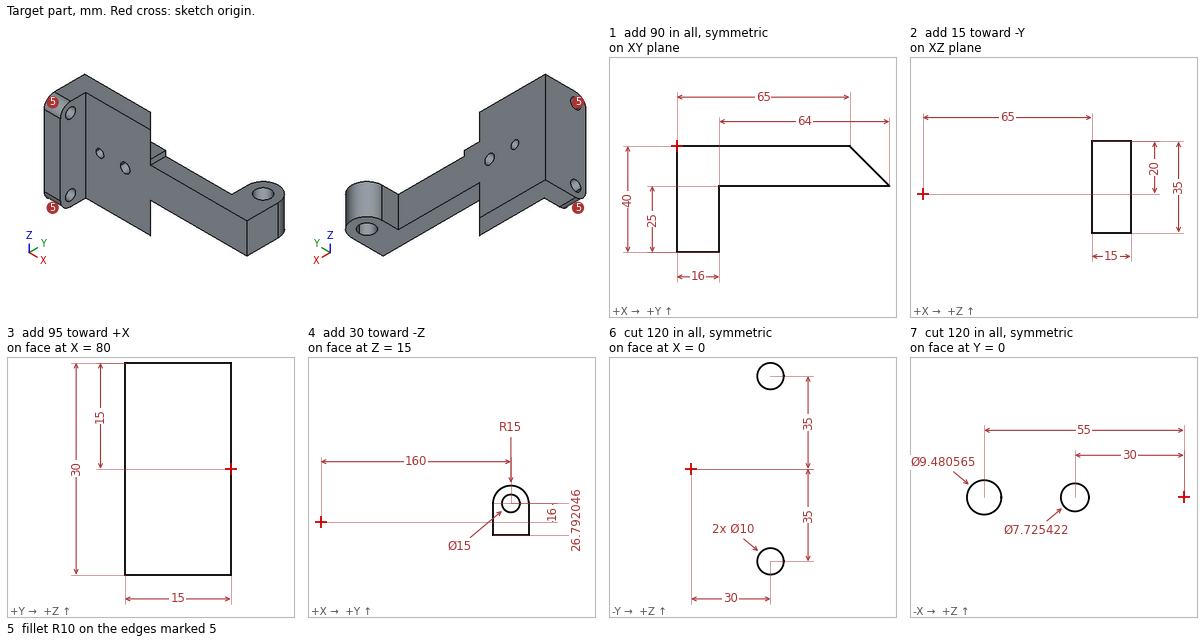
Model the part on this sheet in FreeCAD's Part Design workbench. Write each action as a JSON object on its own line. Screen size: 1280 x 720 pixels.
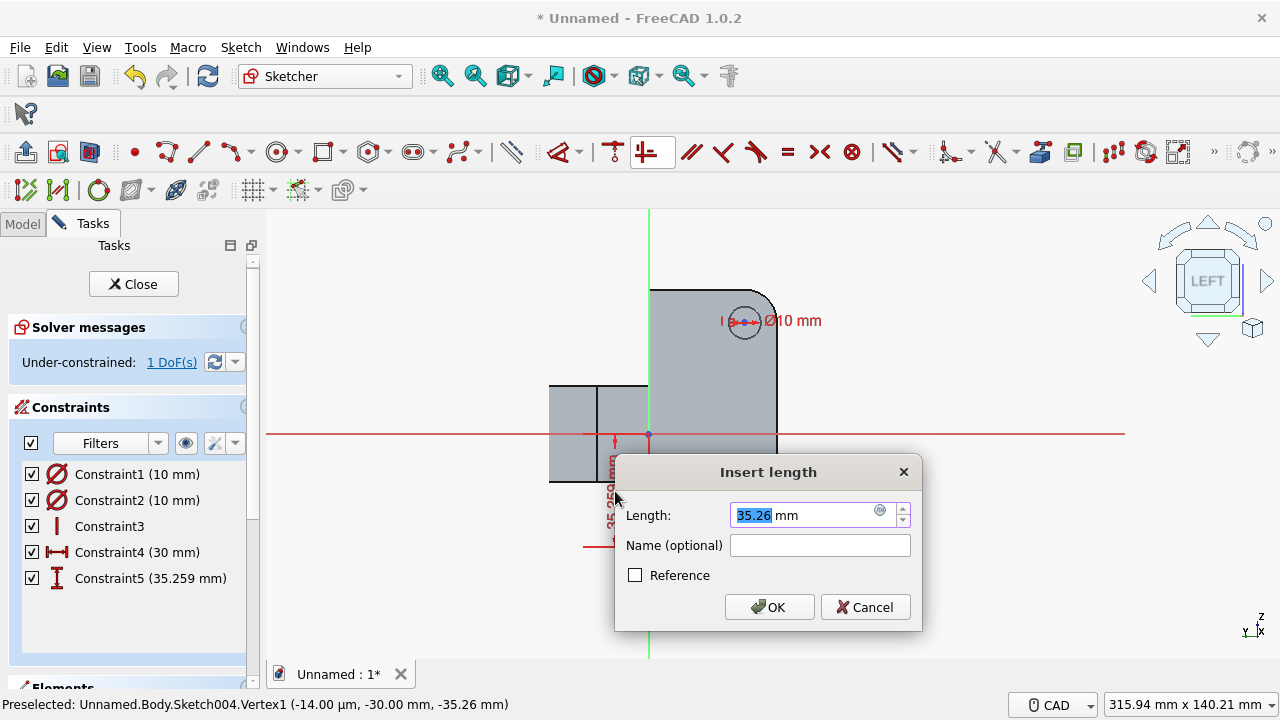
{"action": "type", "text": "35"}
{"action": "key", "text": "Return"}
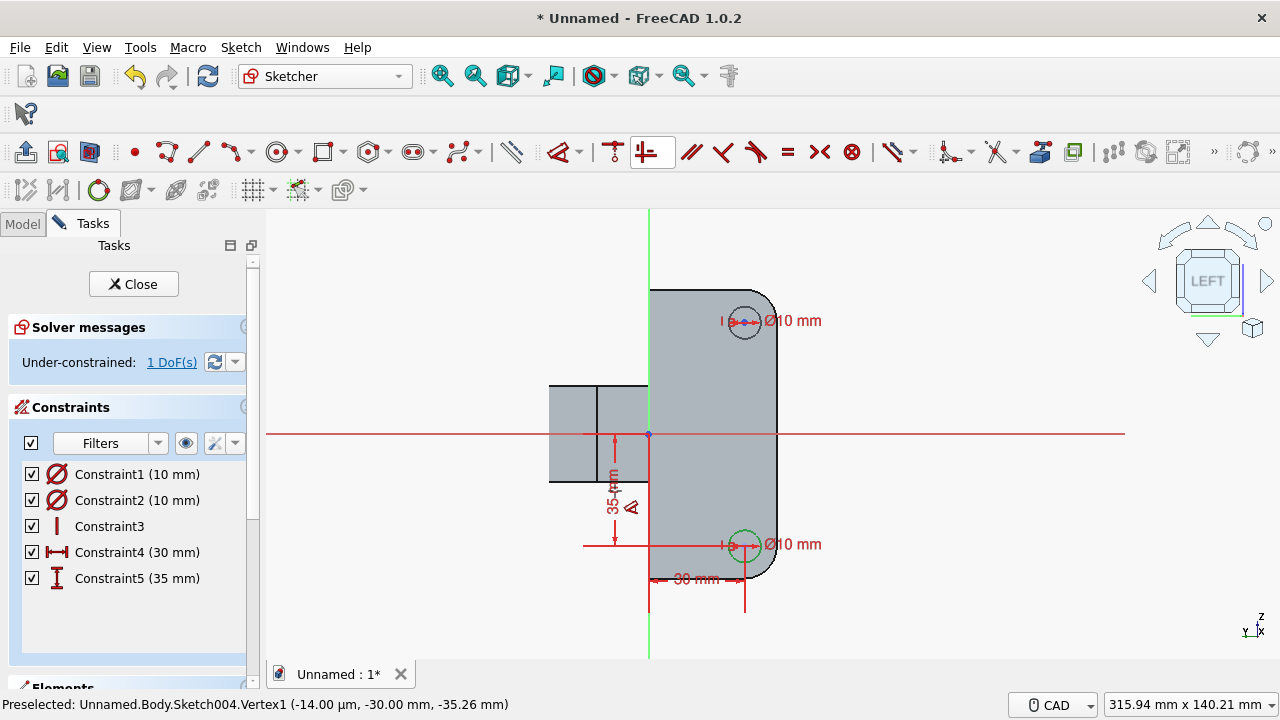
{"action": "left_click", "coordinate": [745, 323]}
{"action": "left_click", "coordinate": [615, 378]}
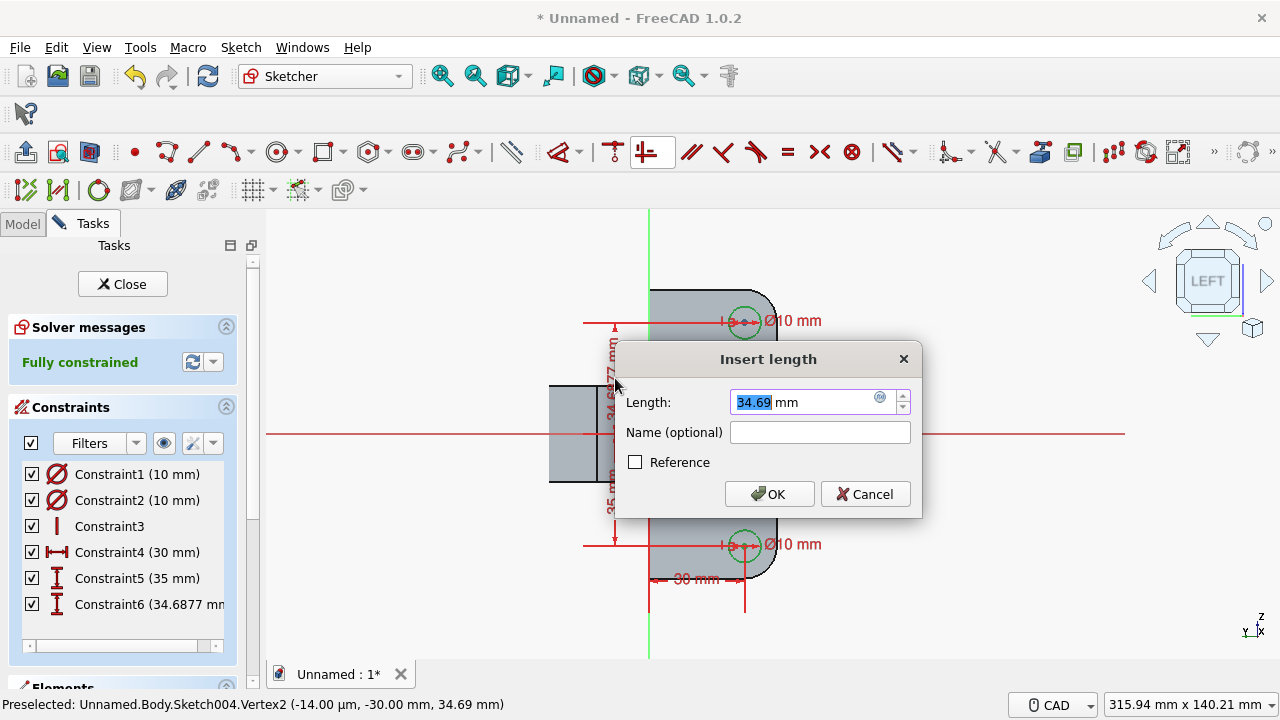
{"action": "type", "text": "35"}
{"action": "key", "text": "Return"}
{"action": "key", "text": "Escape"}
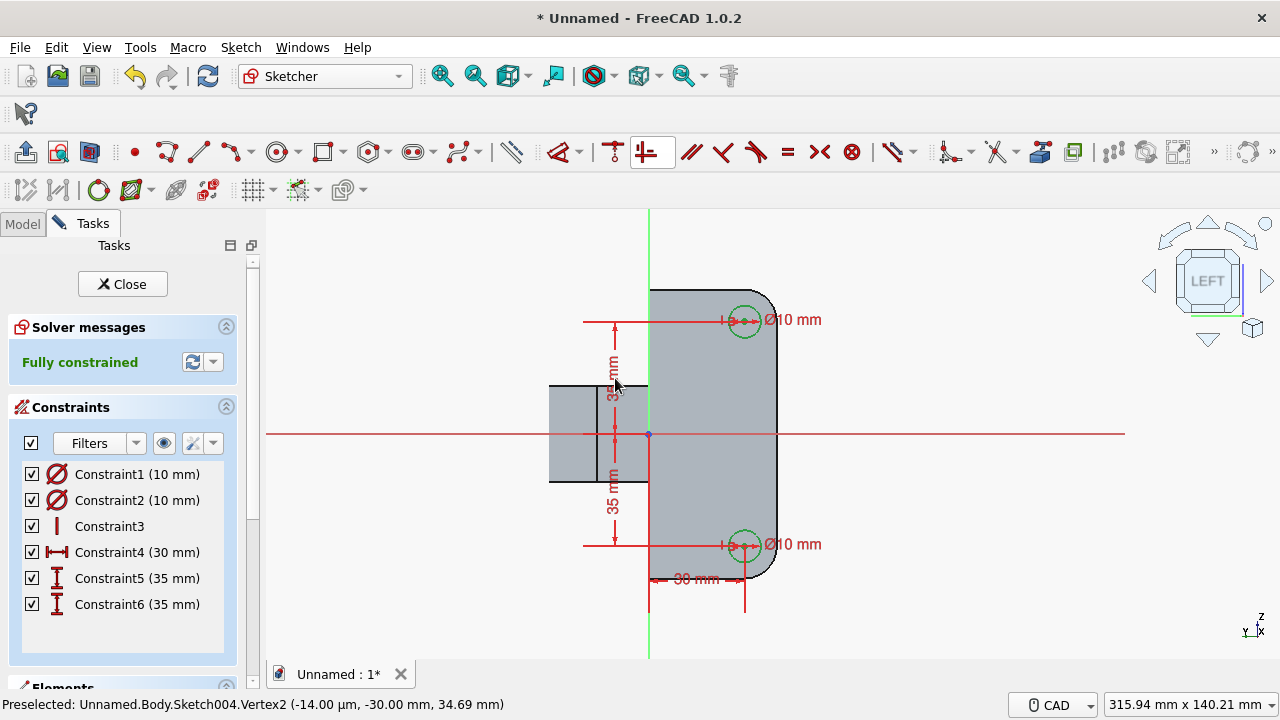
{"action": "left_click", "coordinate": [123, 284]}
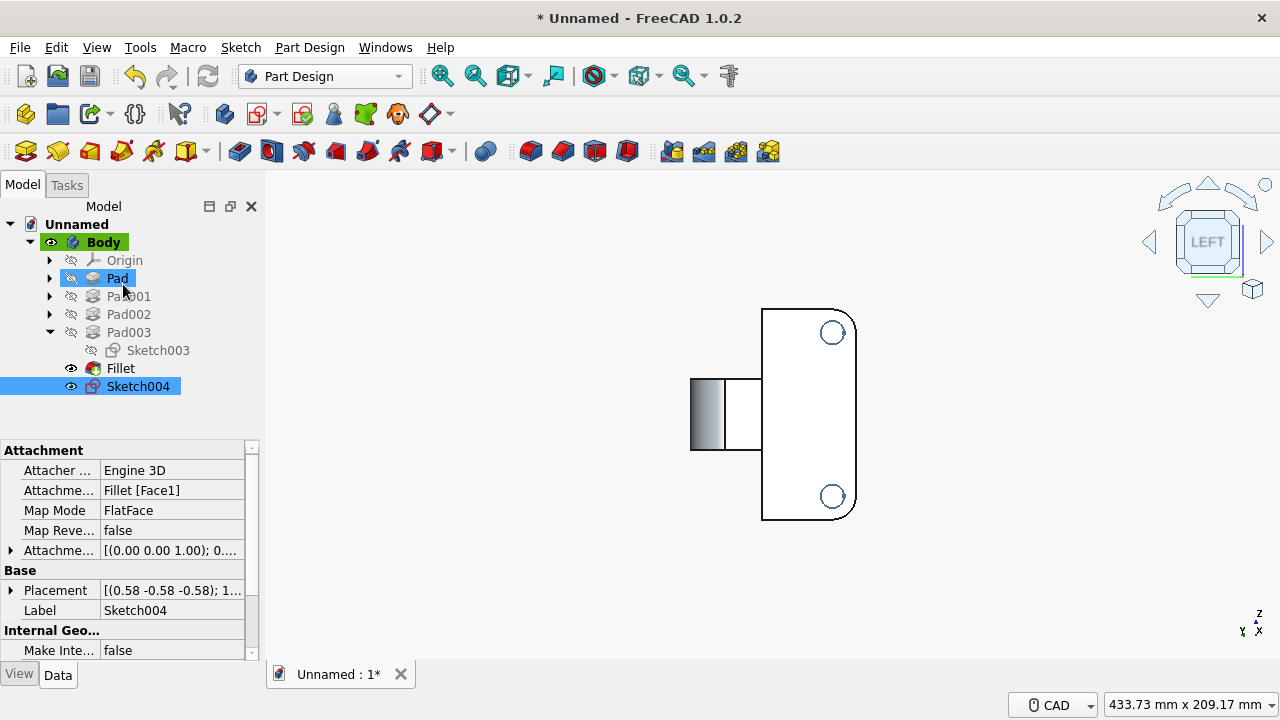
{"action": "left_click", "coordinate": [240, 152]}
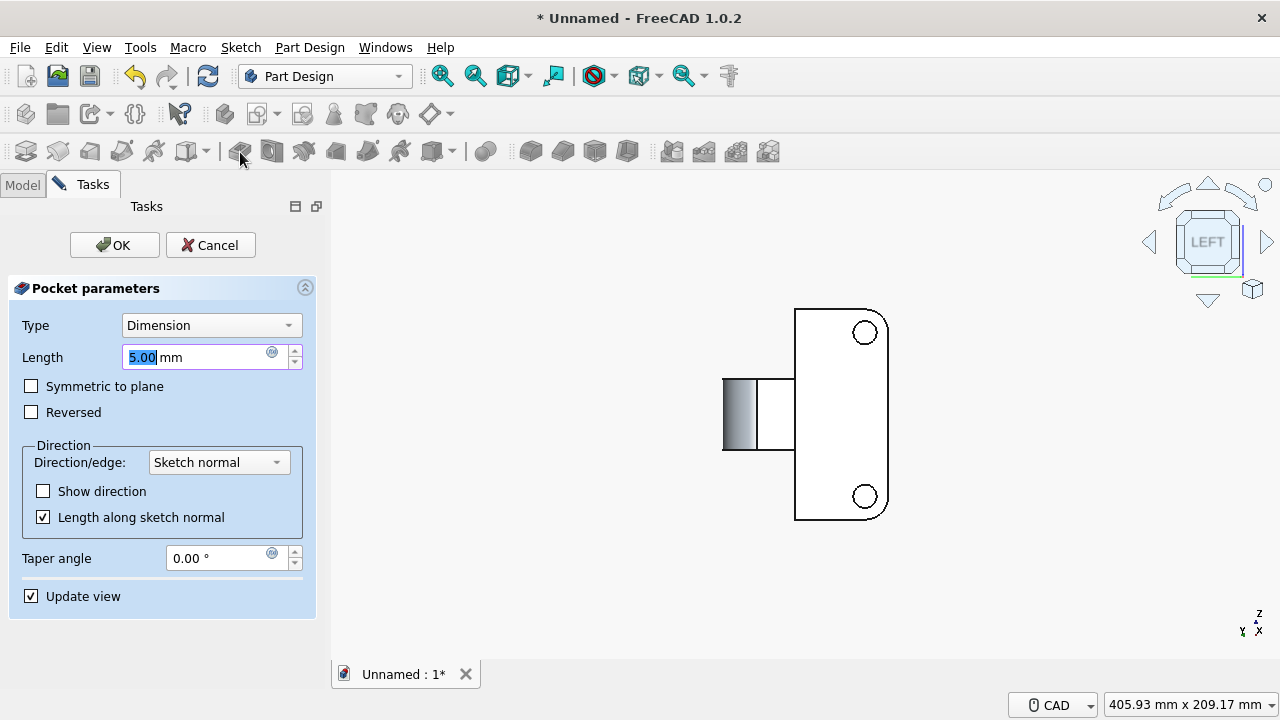
{"action": "type", "text": "120"}
{"action": "key", "text": "Tab"}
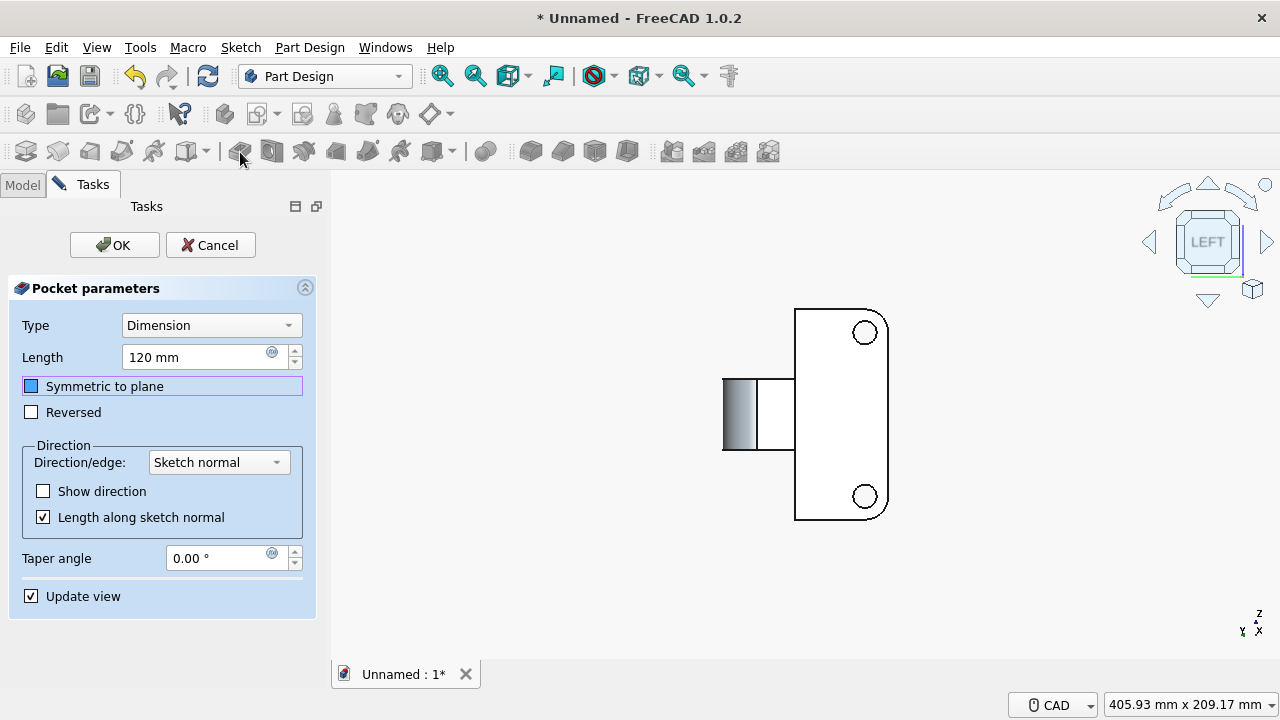
{"action": "left_click", "coordinate": [30, 386]}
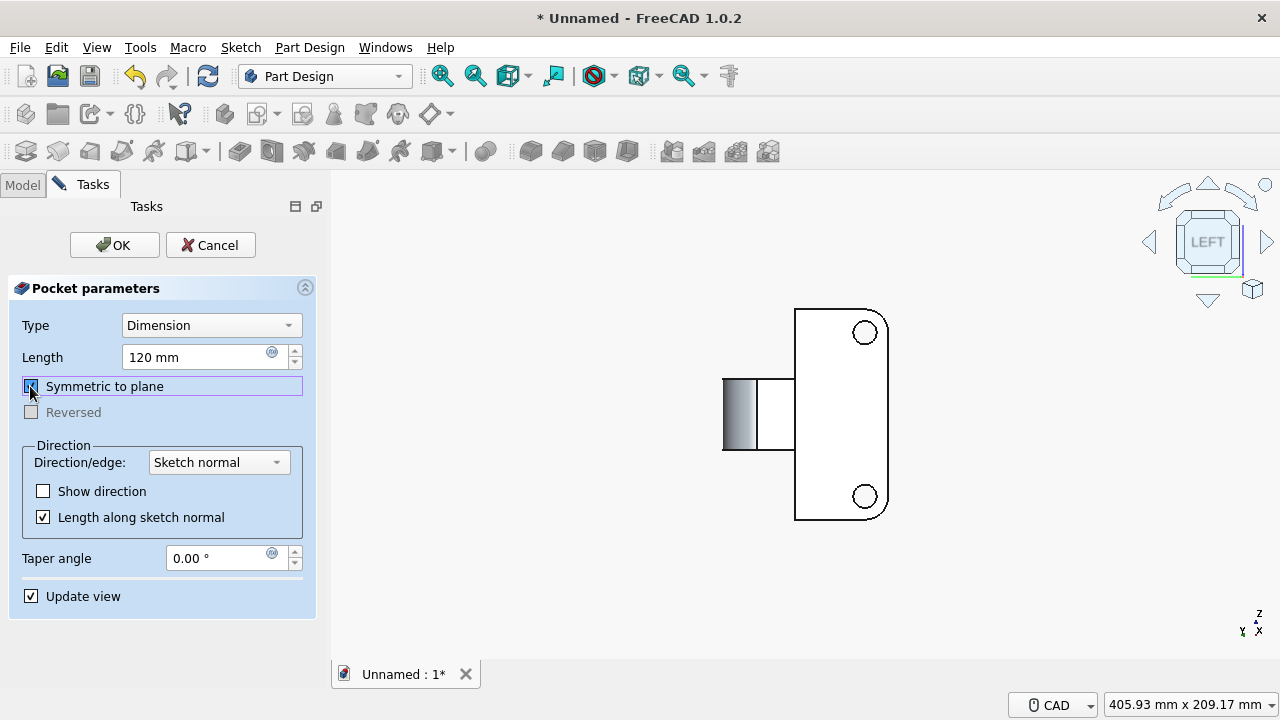
{"action": "left_click", "coordinate": [115, 245]}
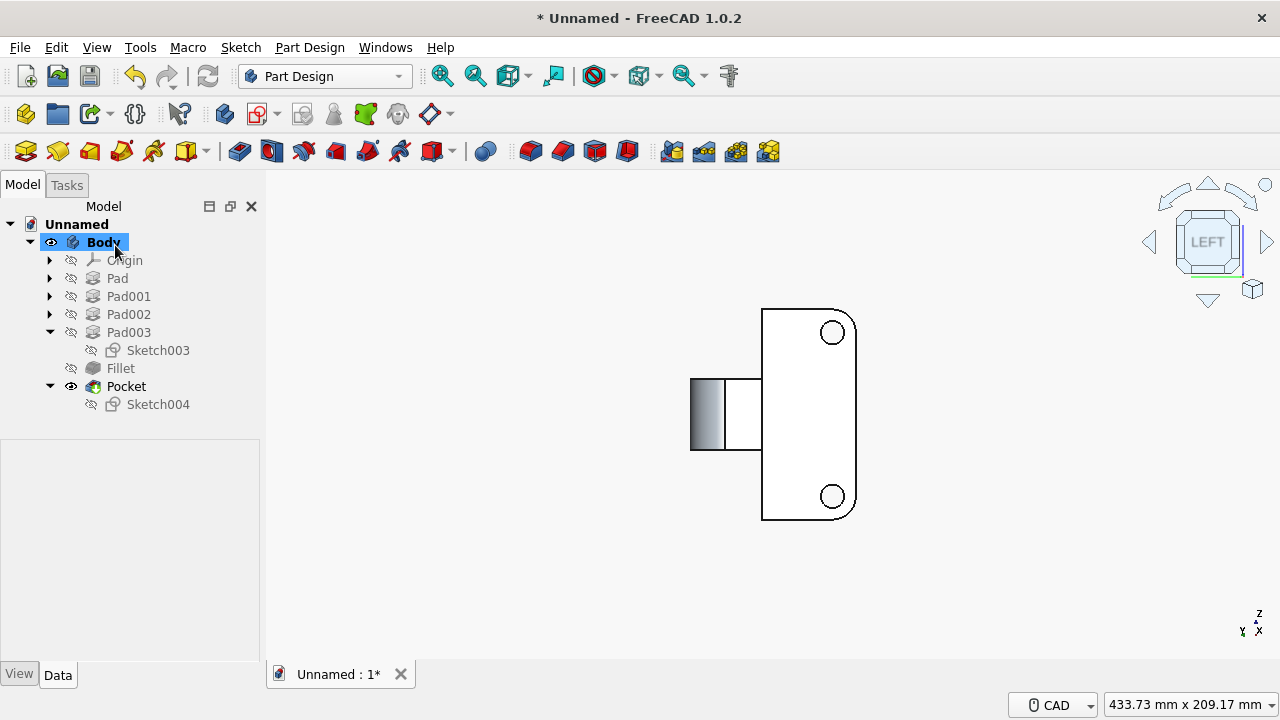
{"action": "key", "text": "v f"}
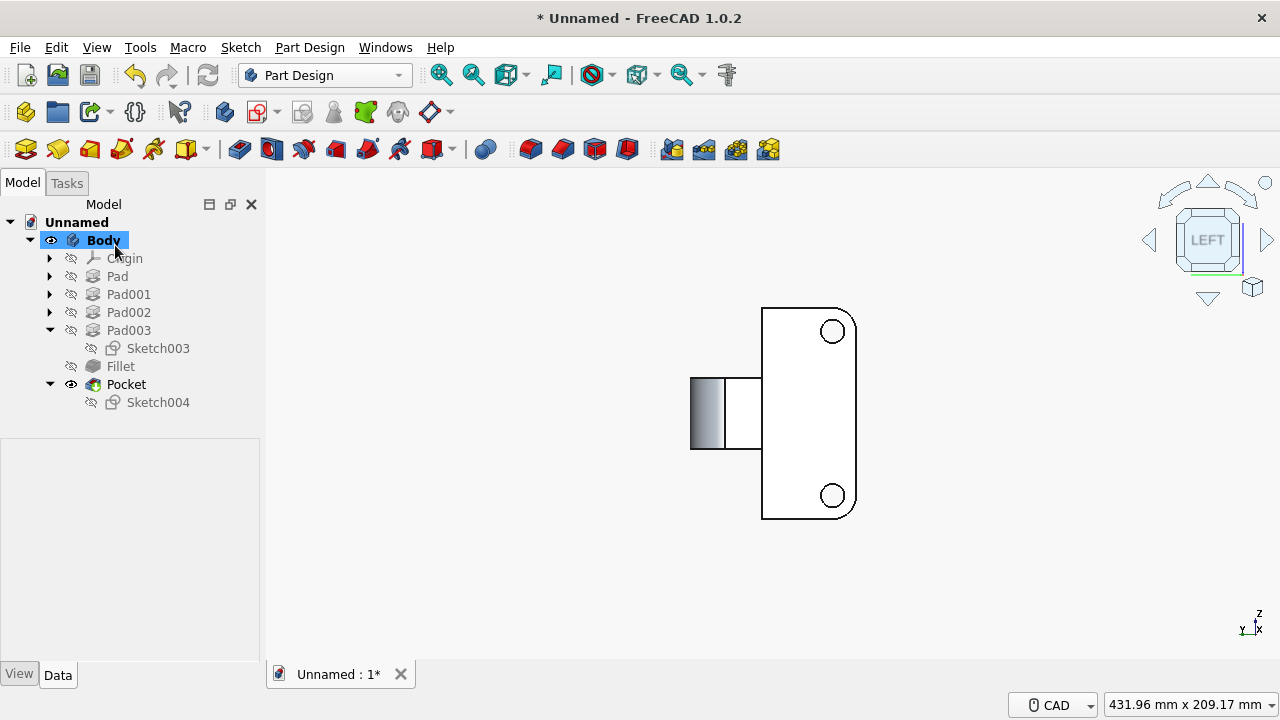
{"action": "key", "text": "4"}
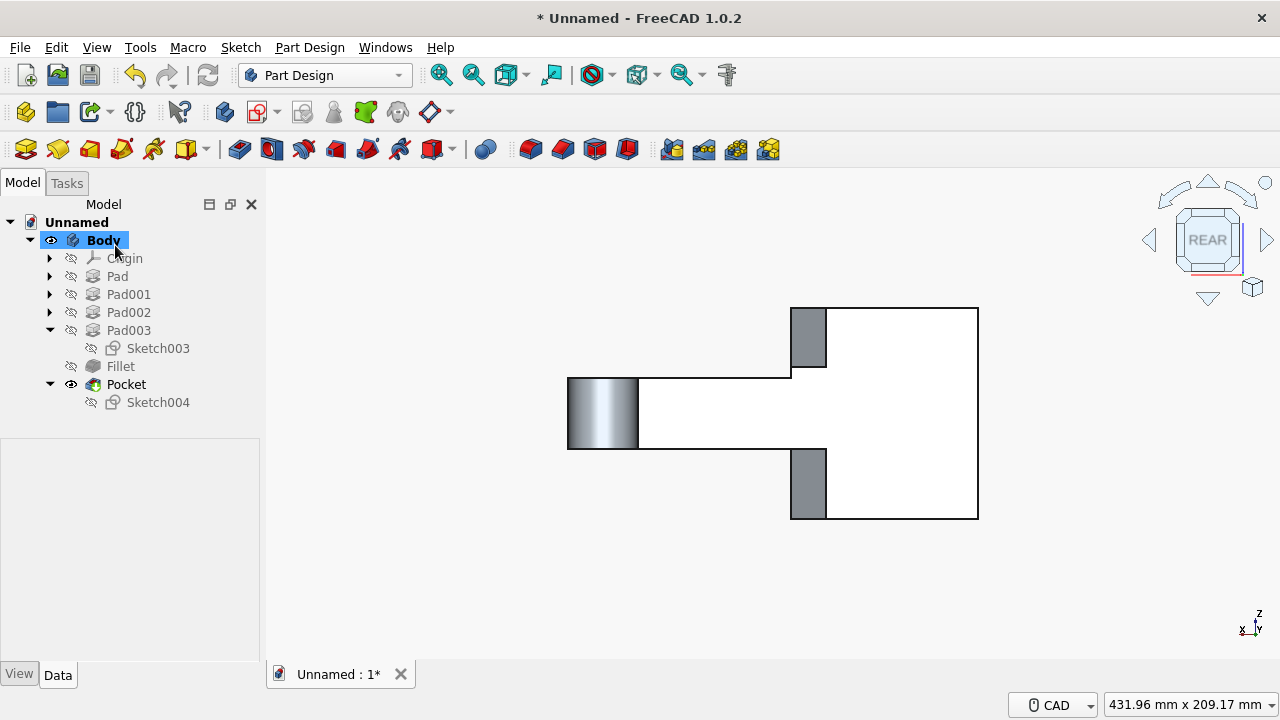
{"action": "left_click", "coordinate": [442, 76]}